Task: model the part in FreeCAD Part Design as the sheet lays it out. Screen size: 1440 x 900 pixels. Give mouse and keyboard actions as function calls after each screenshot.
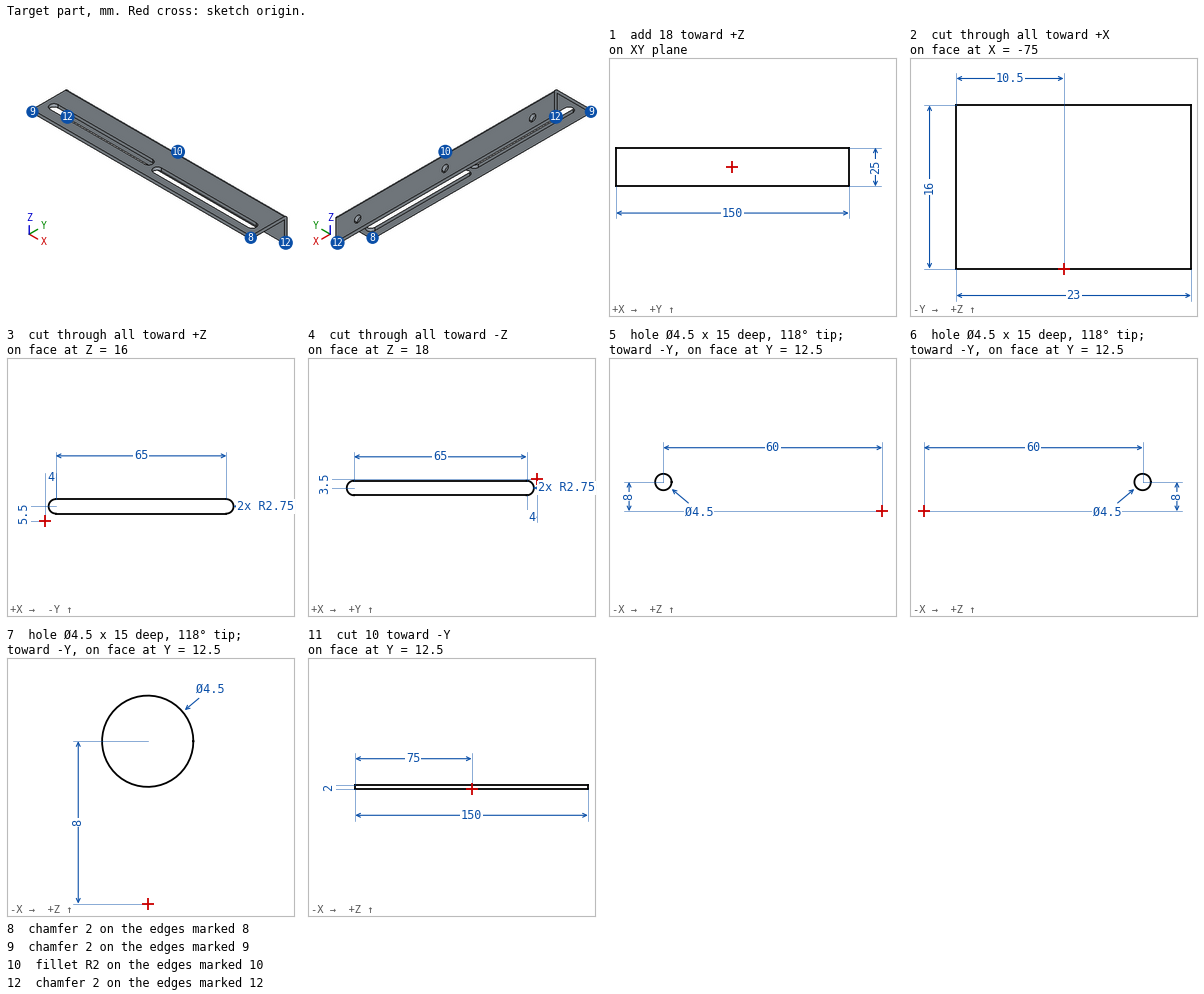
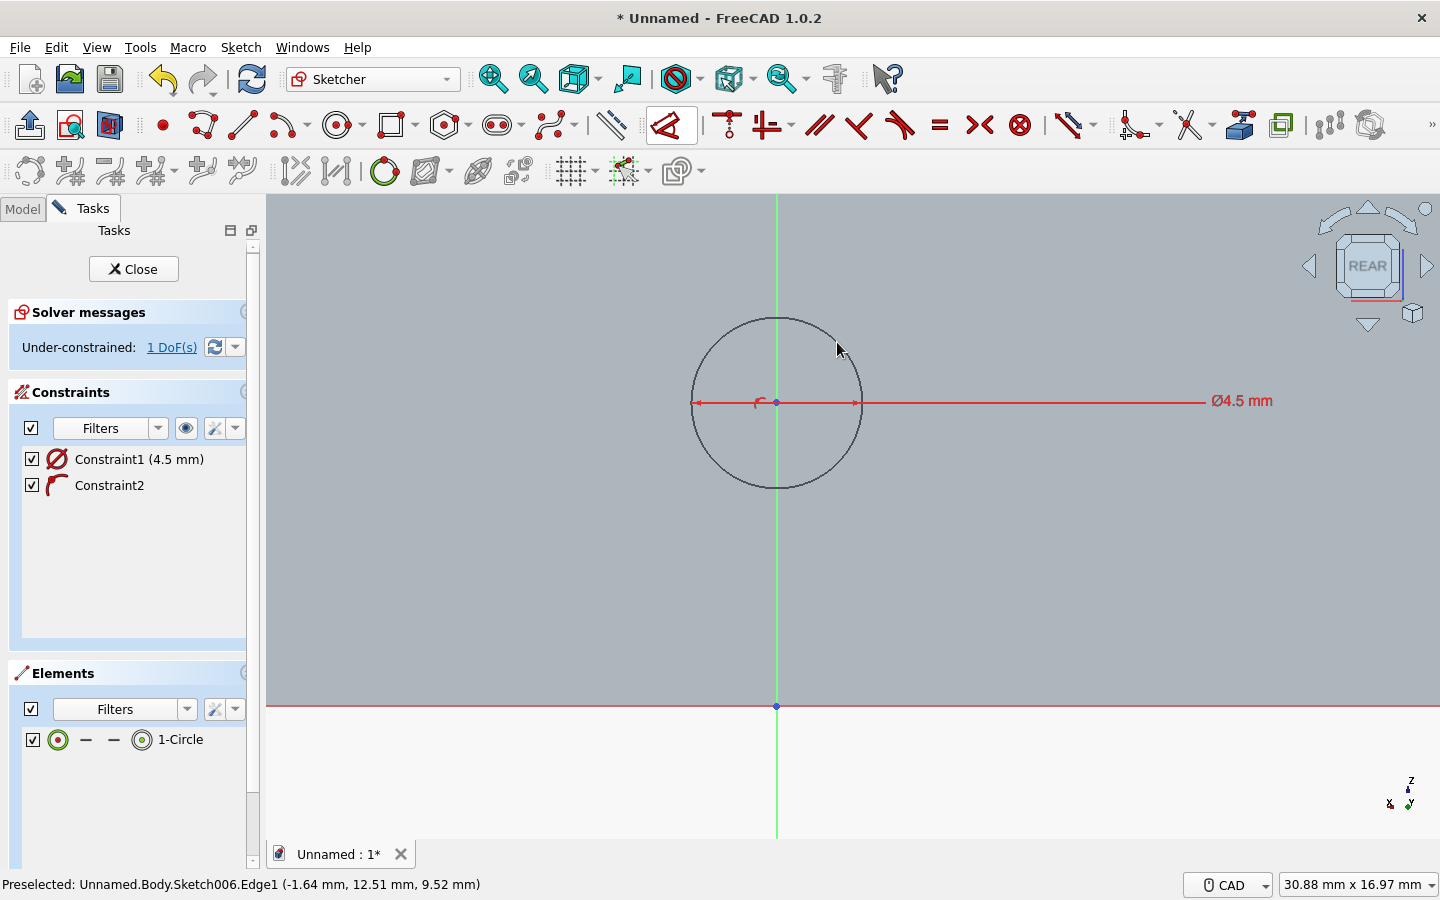
click(777, 403)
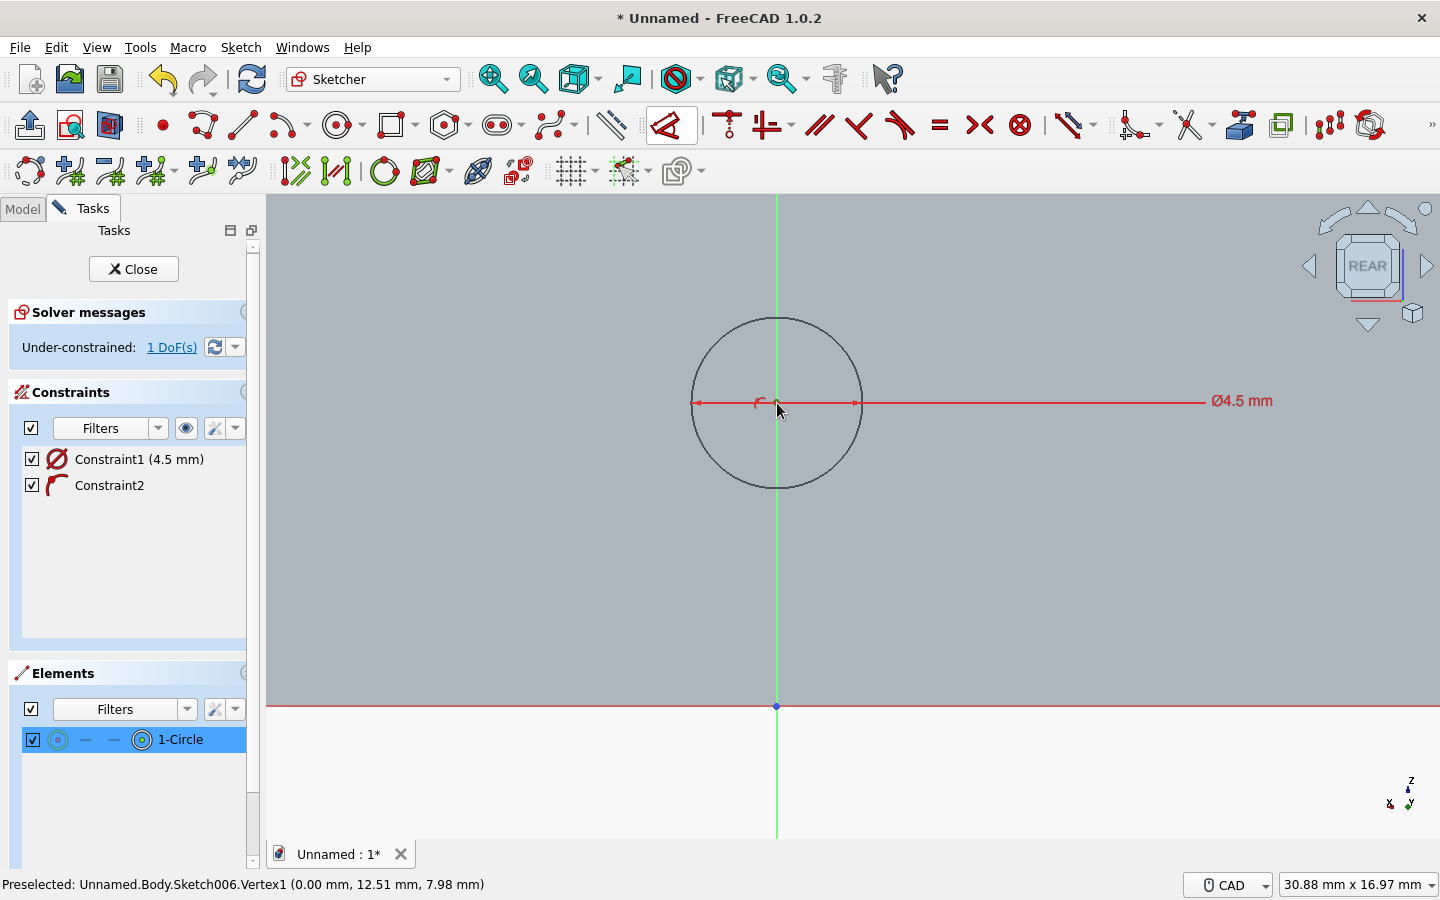
key(i)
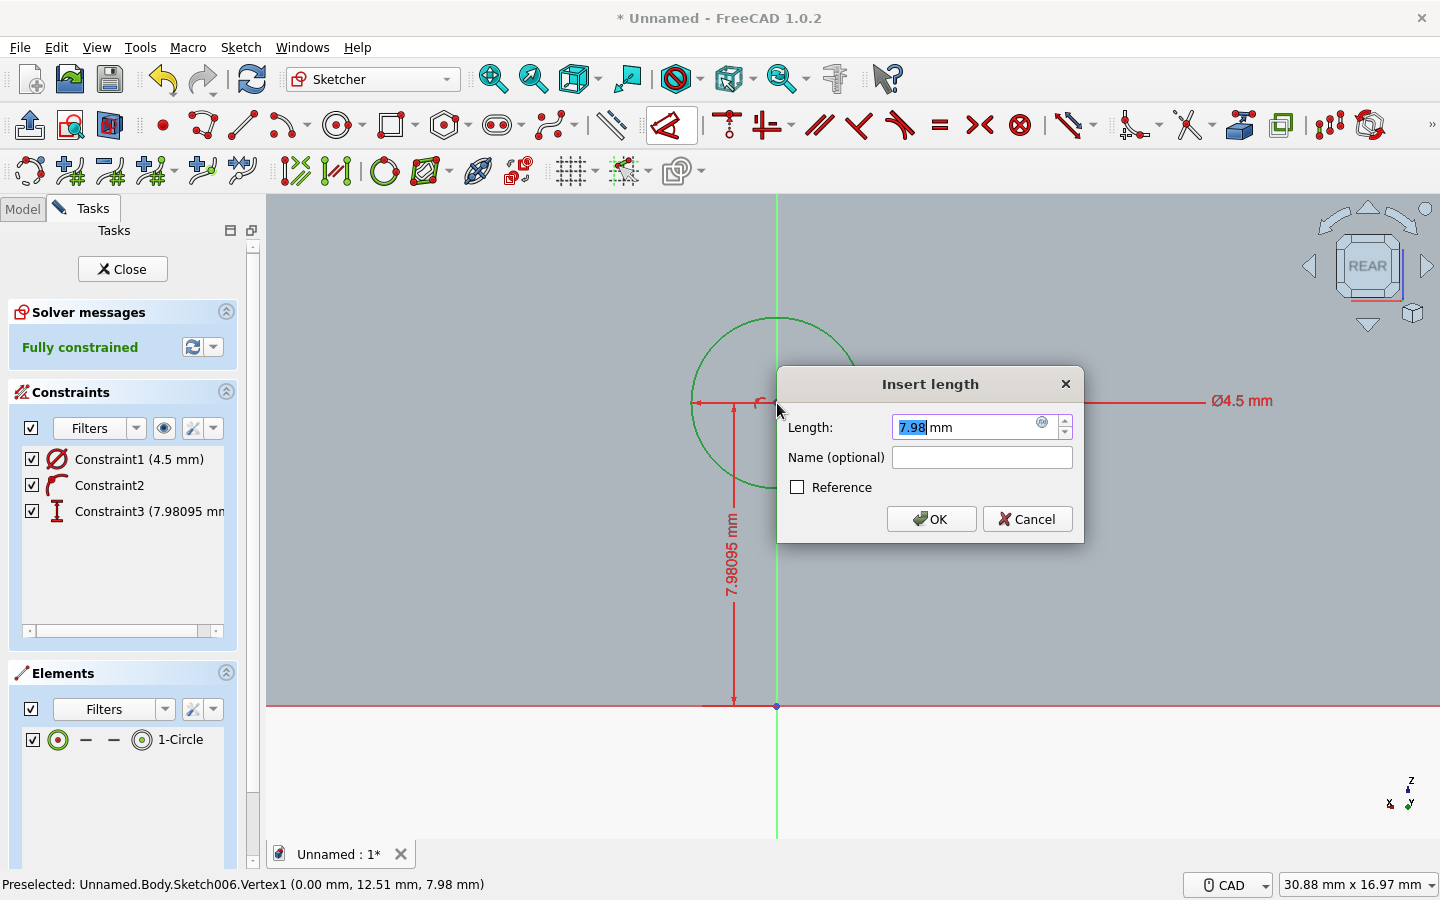
text(8)
key(Return)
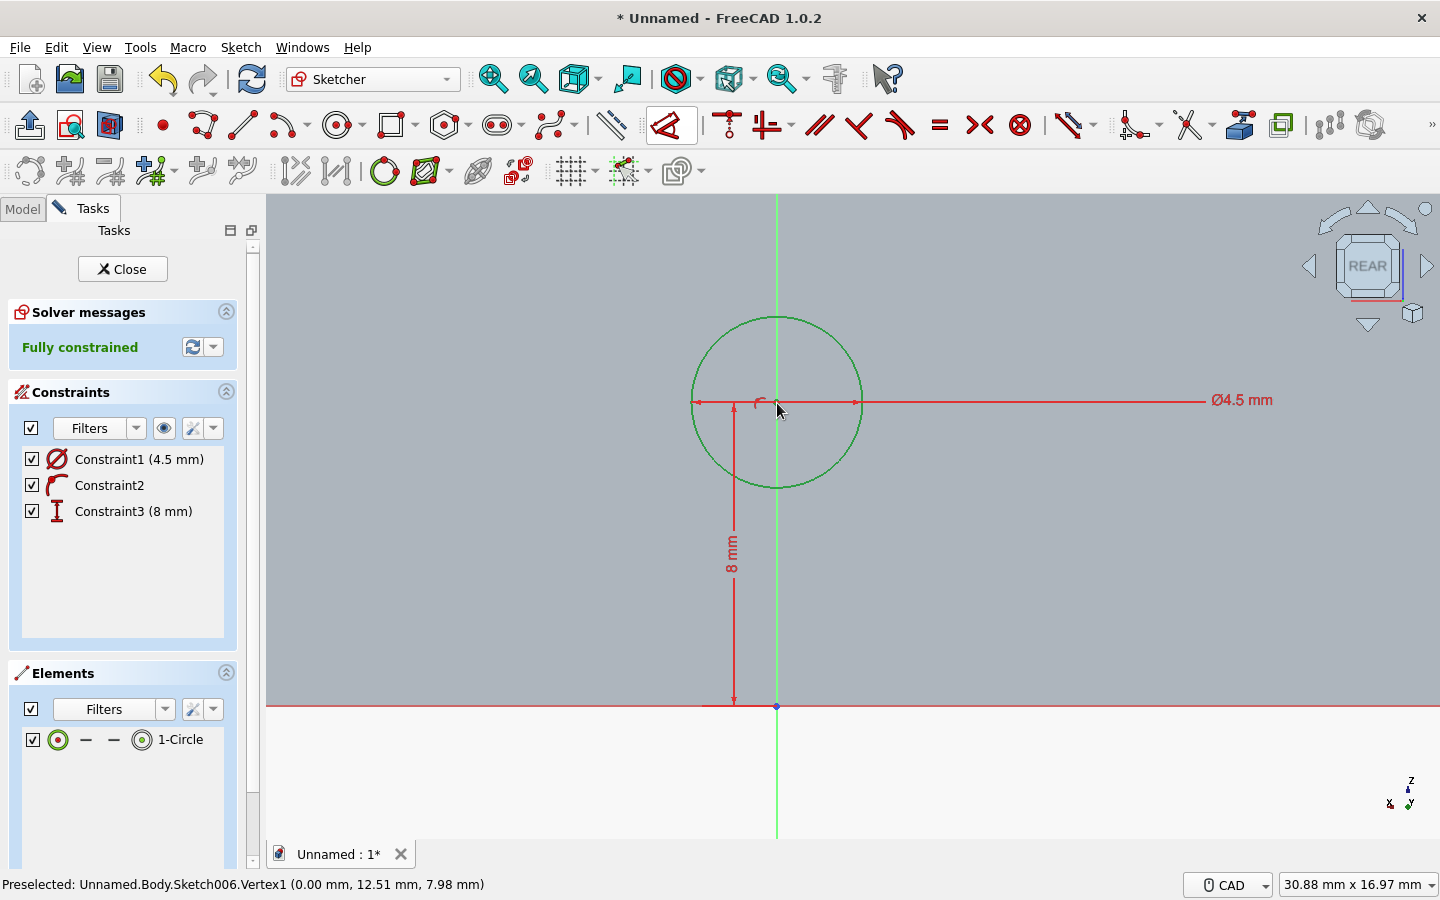
click(123, 269)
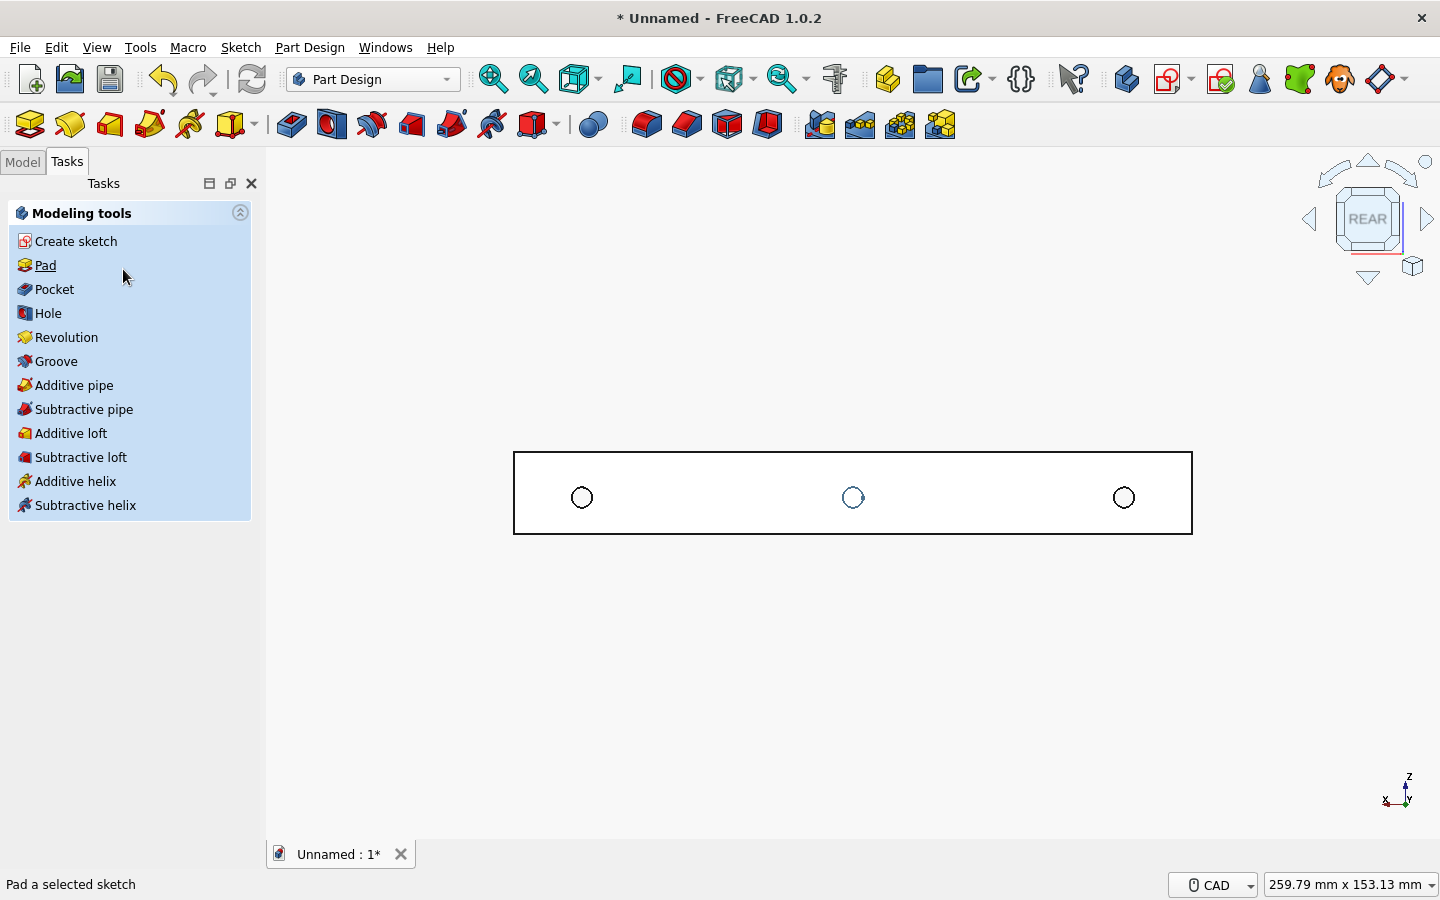
click(332, 124)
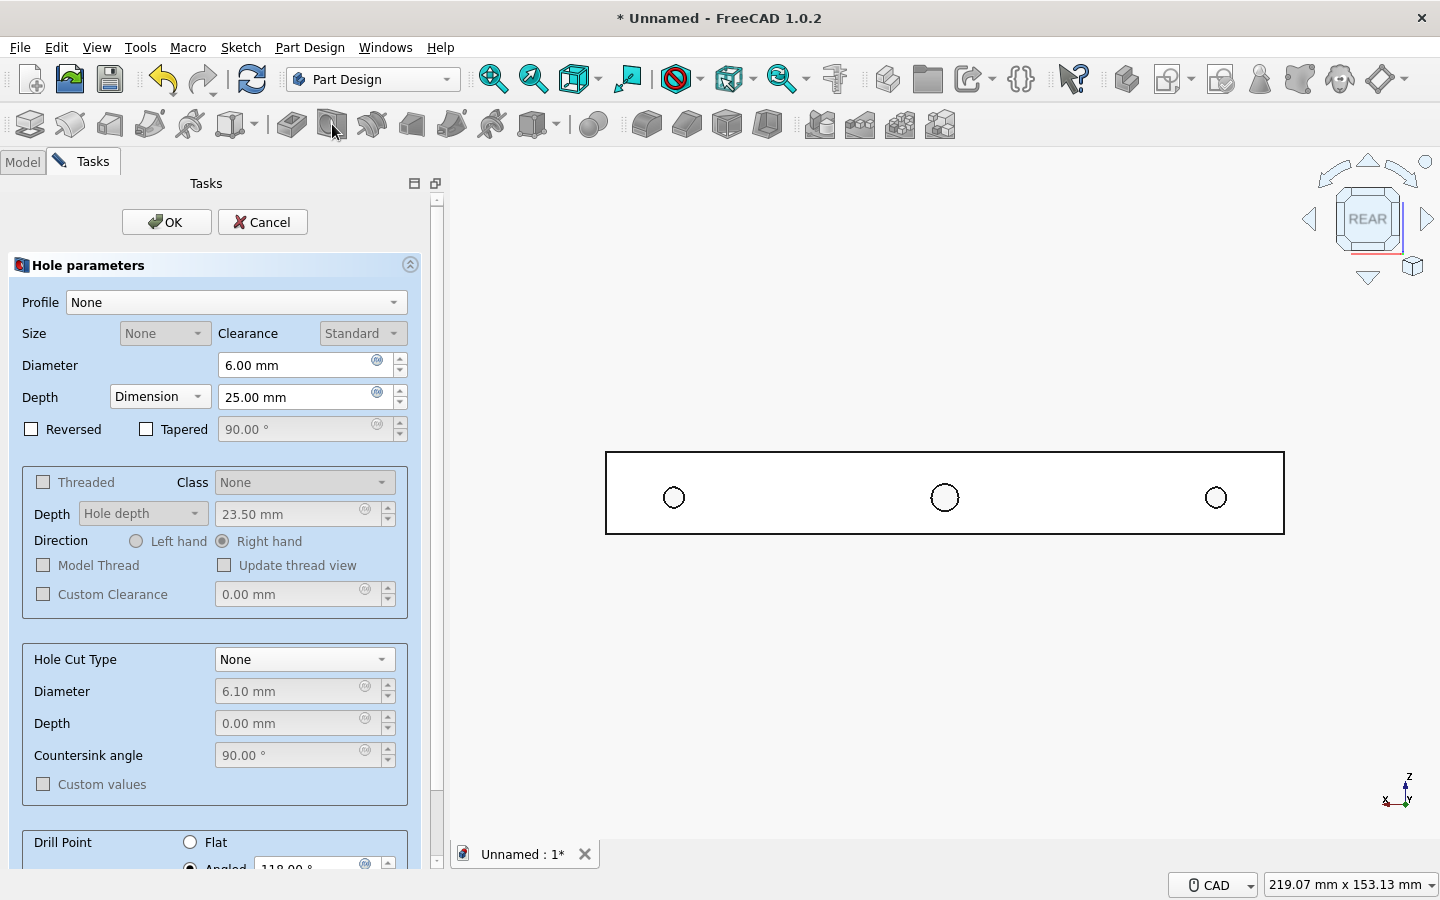
triple_click(305, 365)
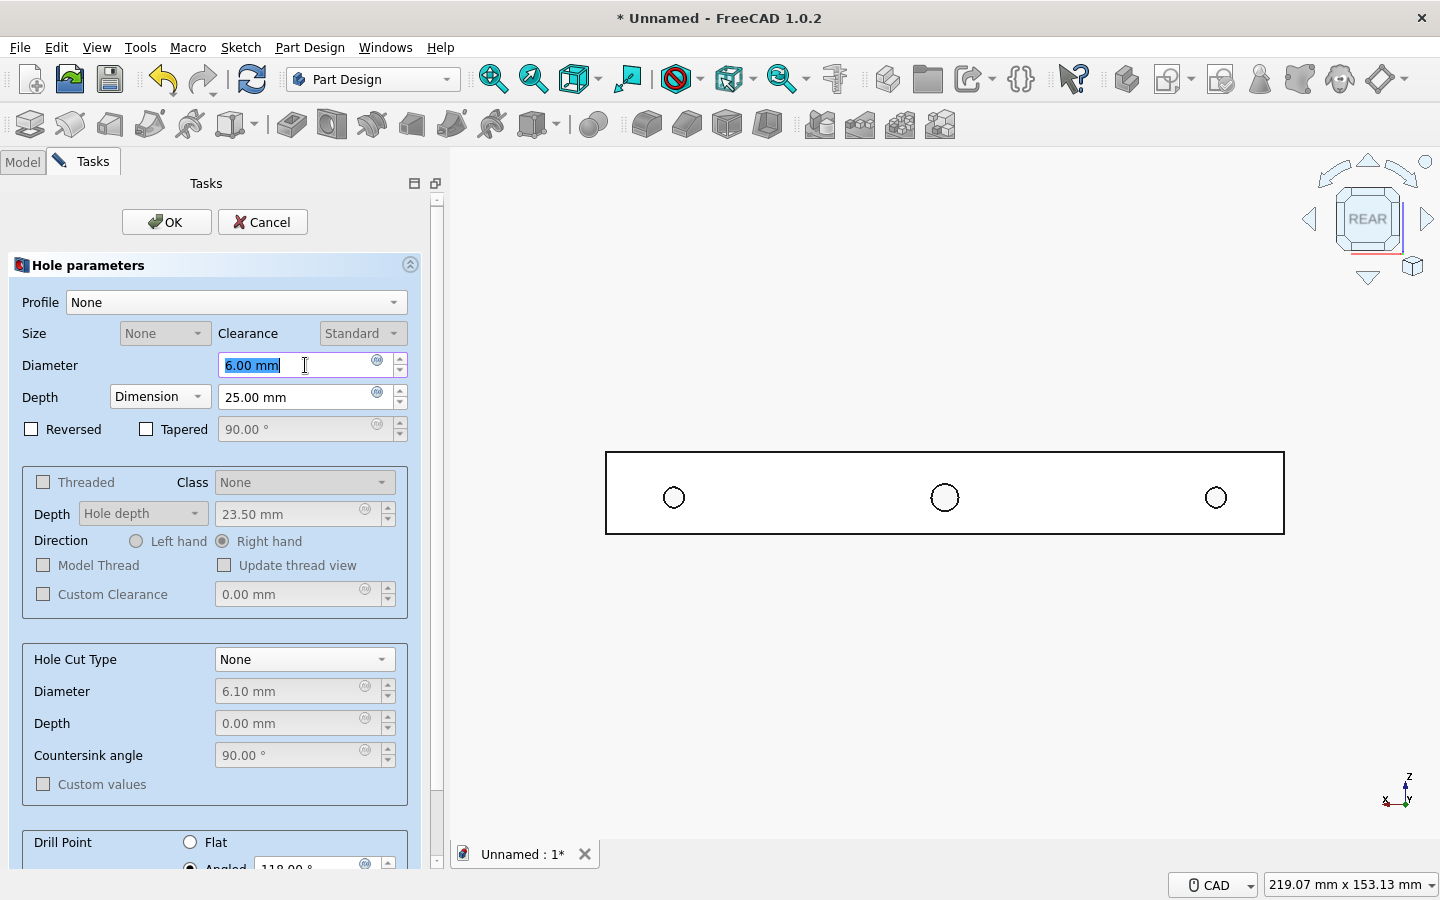
text(4.5)
key(Tab)